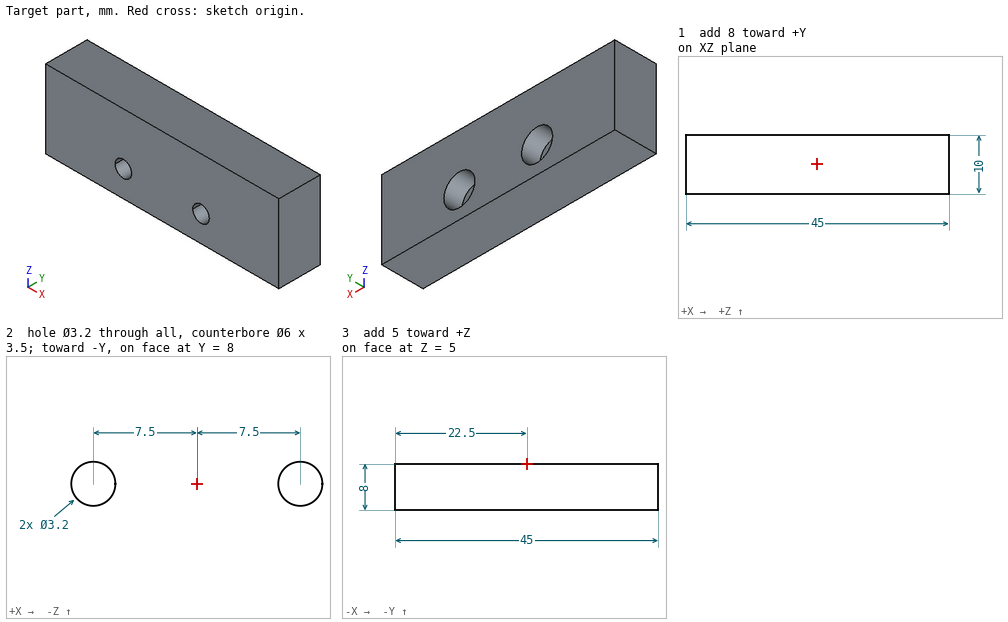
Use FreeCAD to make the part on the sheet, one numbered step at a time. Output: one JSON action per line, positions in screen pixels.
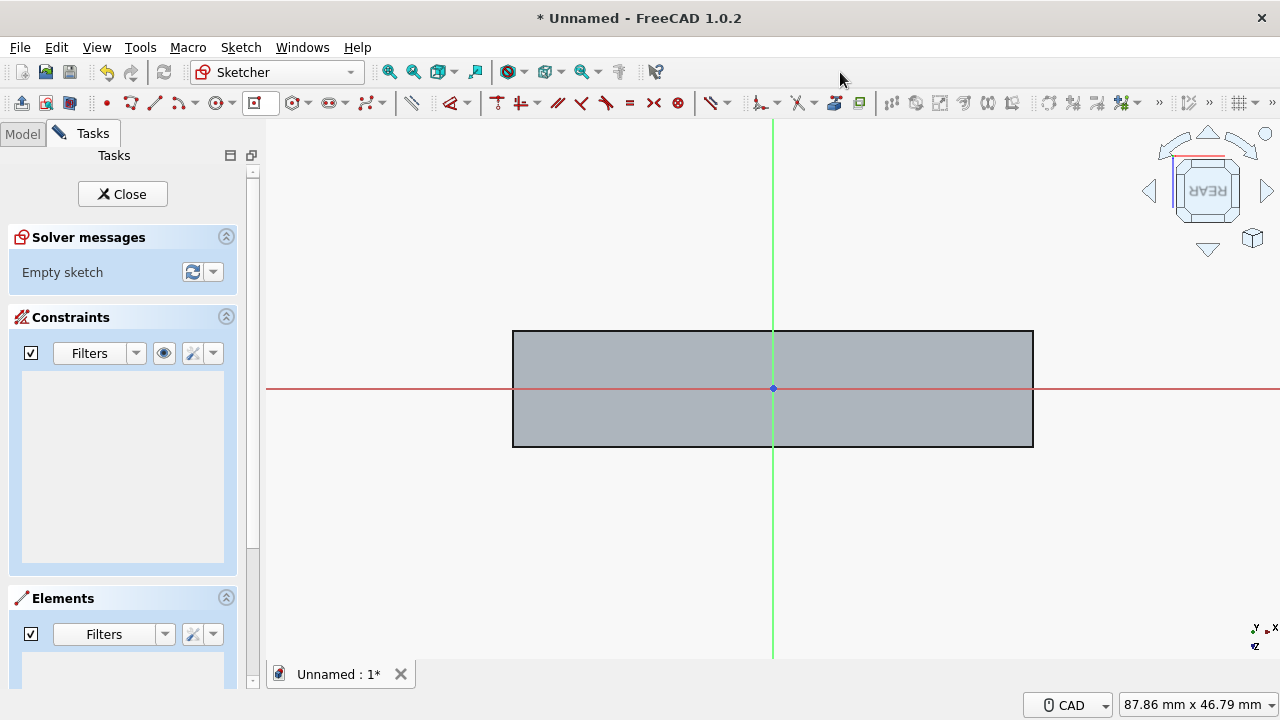
{"action": "scroll", "coordinate": [813, 389], "scroll_direction": "up", "scroll_amount": 5}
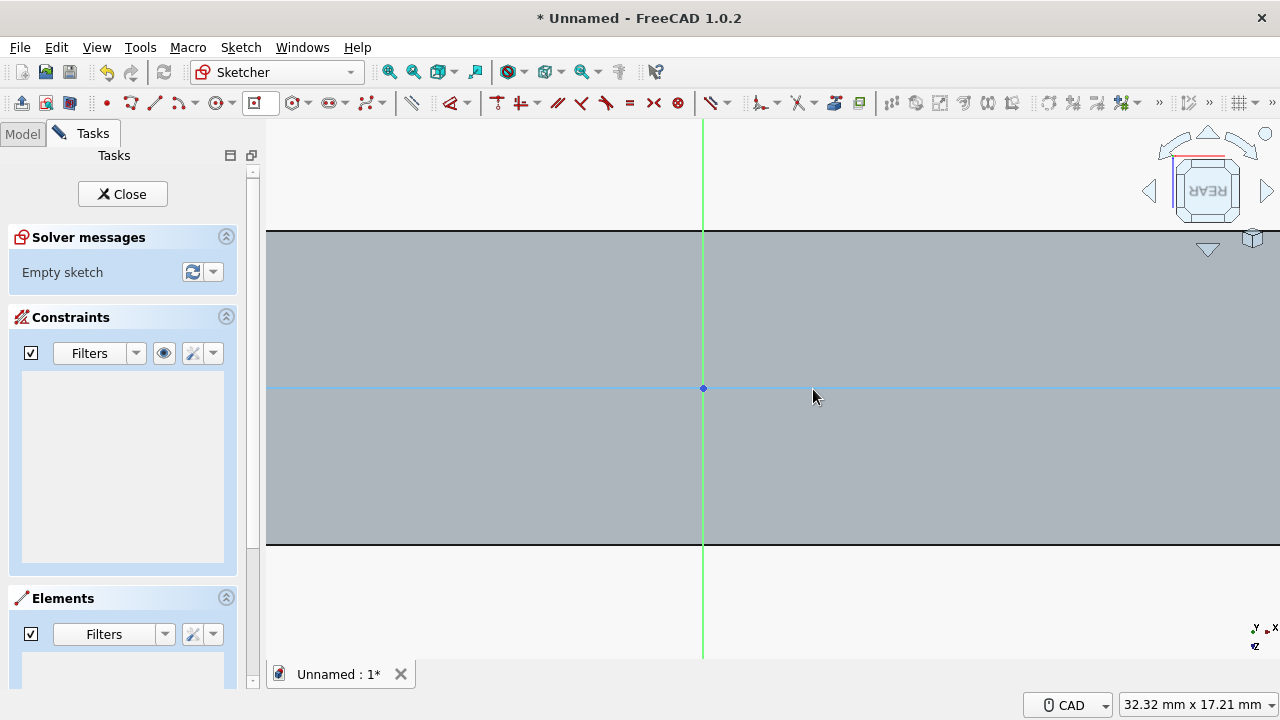
{"action": "key", "text": "g c"}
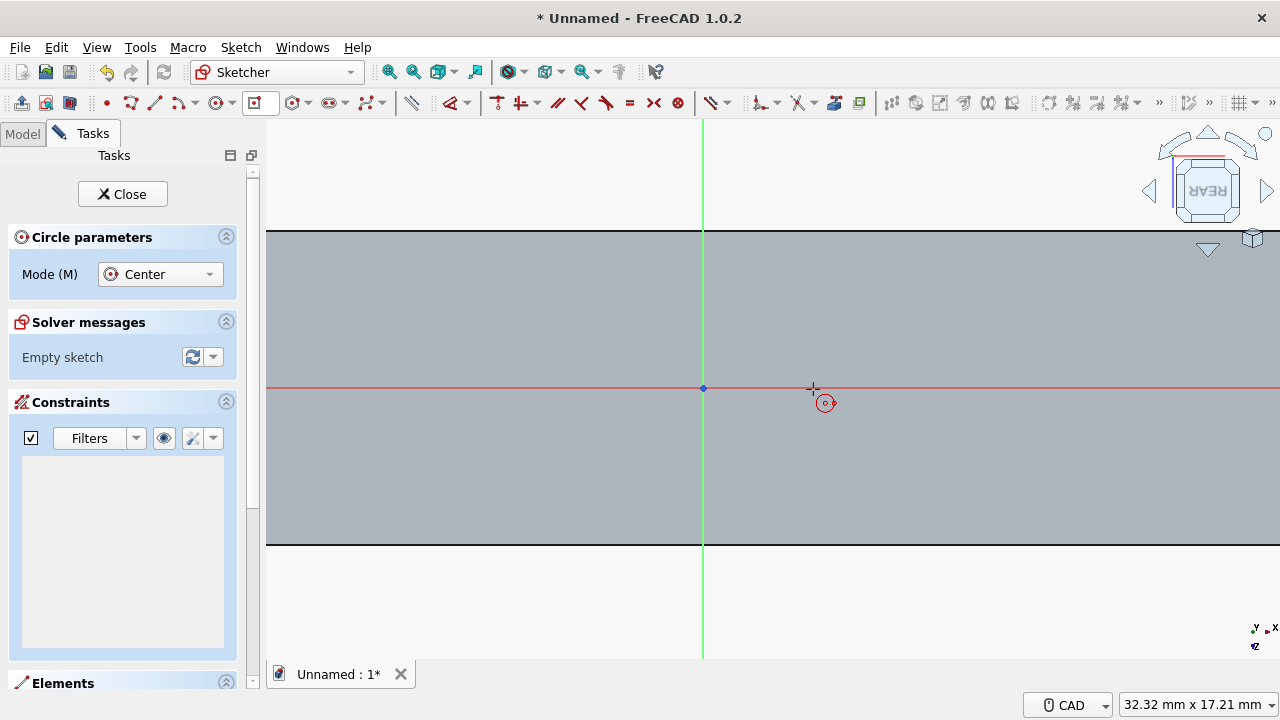
{"action": "left_click", "coordinate": [468, 388]}
{"action": "left_click", "coordinate": [504, 353]}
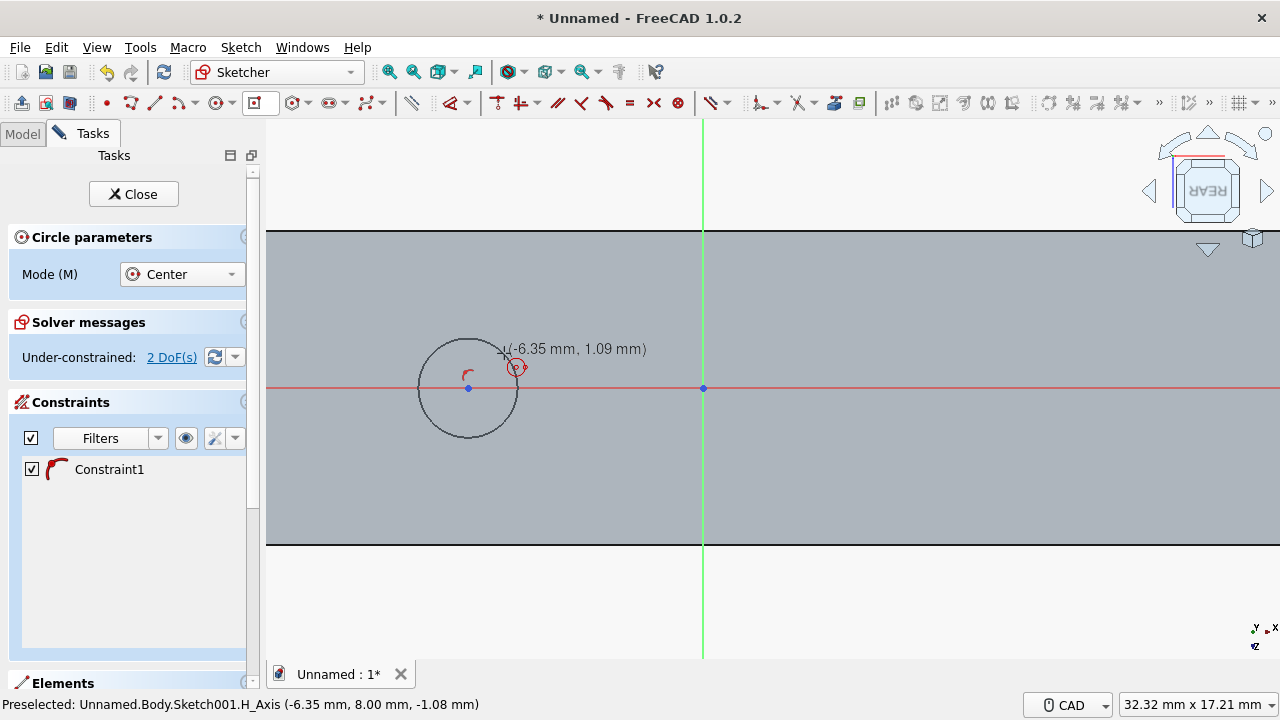
{"action": "left_click", "coordinate": [939, 388]}
{"action": "left_click", "coordinate": [974, 353]}
{"action": "key", "text": "Escape"}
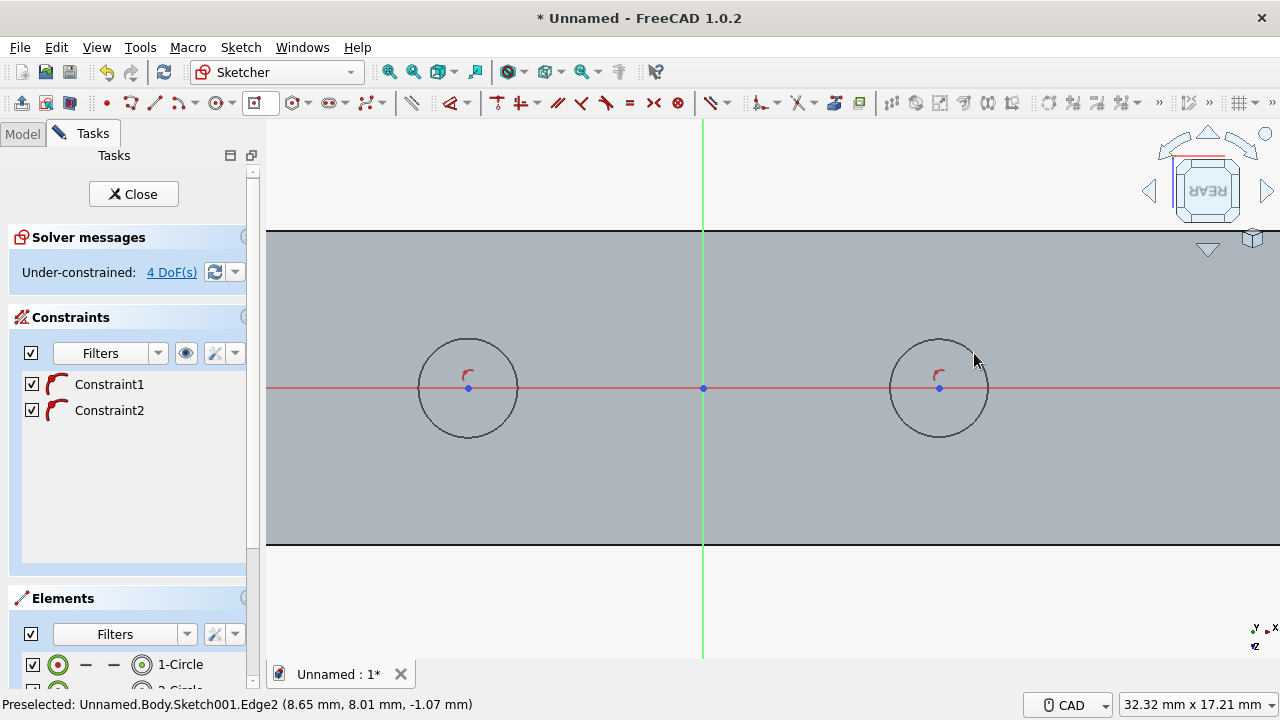
{"action": "left_click", "coordinate": [503, 353]}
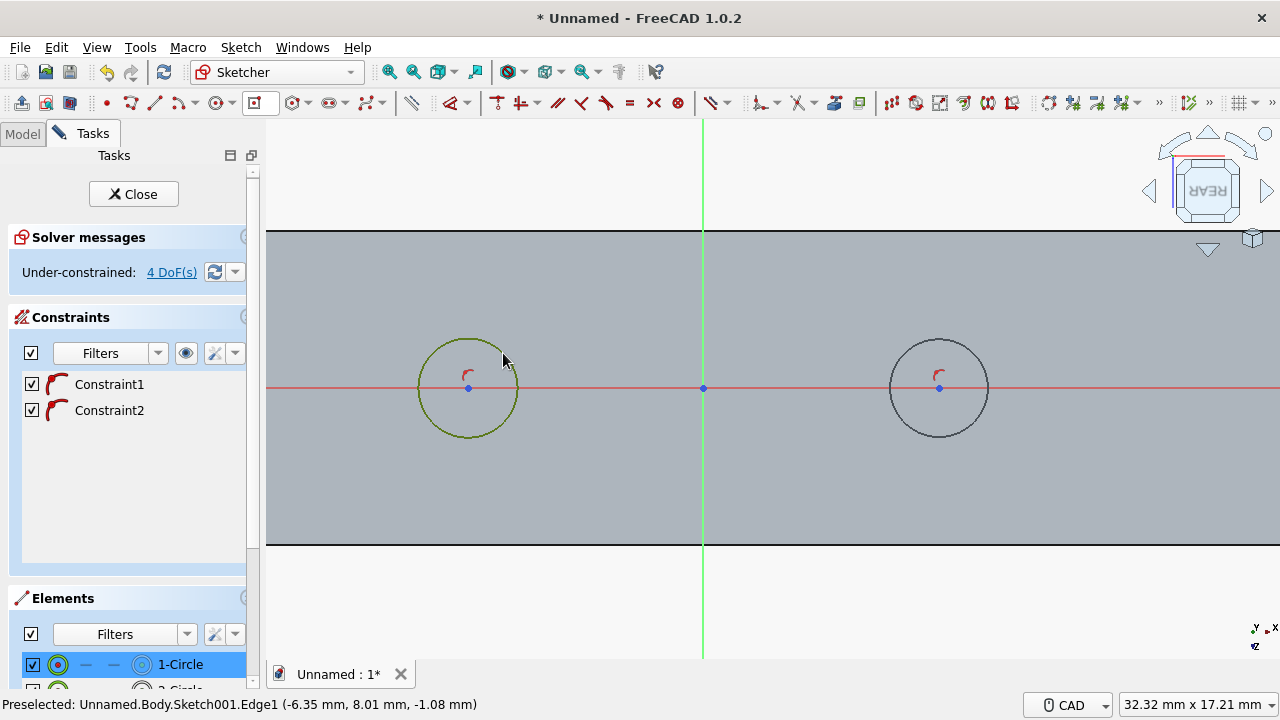
{"action": "left_click", "coordinate": [973, 353]}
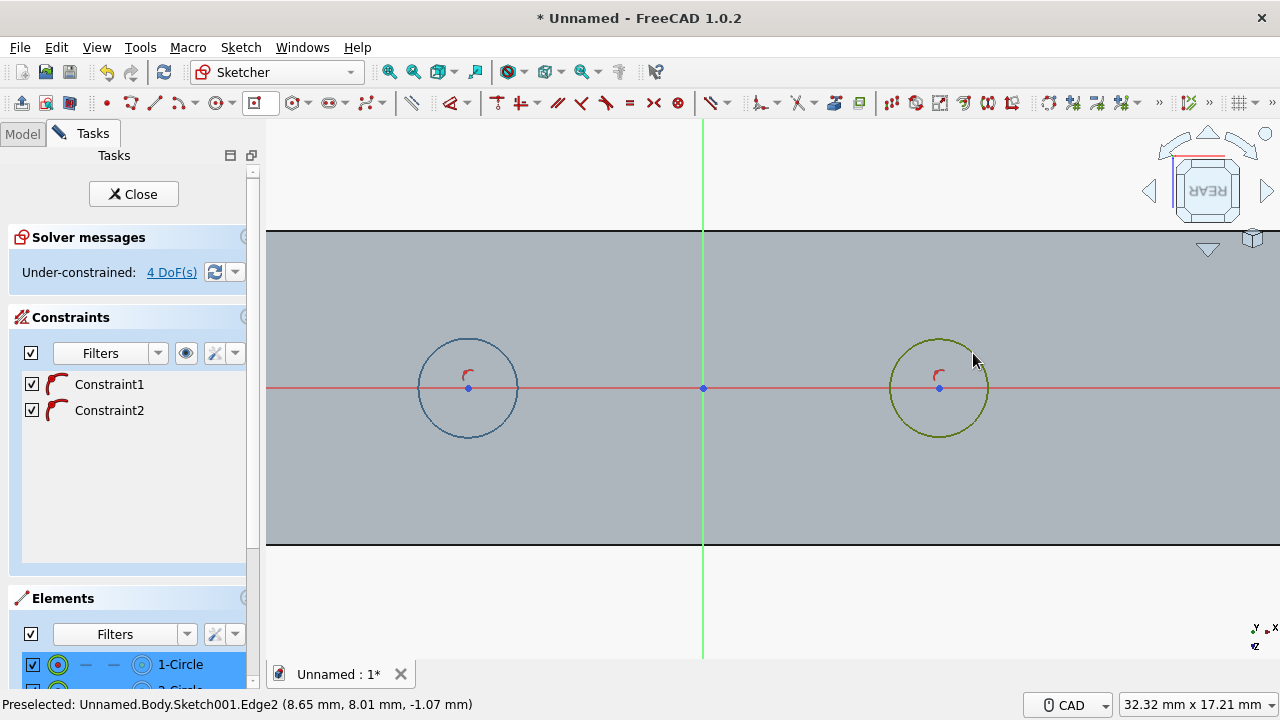
{"action": "left_click", "coordinate": [630, 104]}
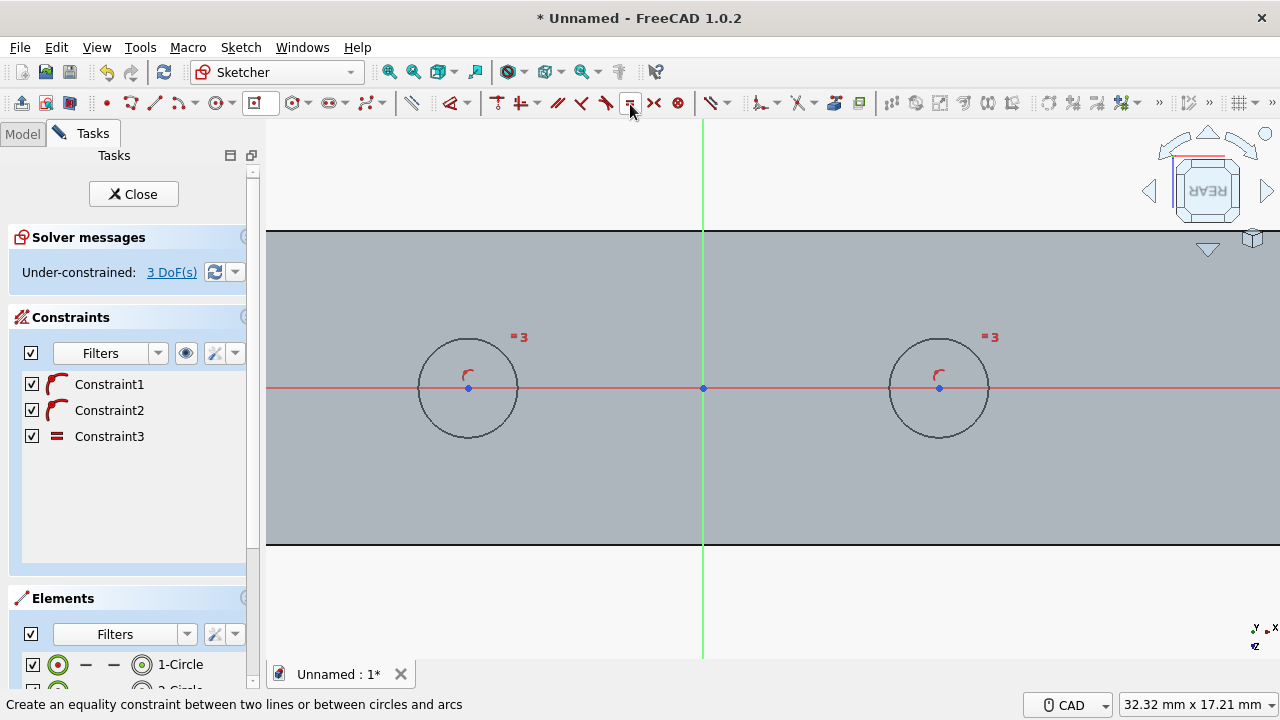
{"action": "left_click", "coordinate": [450, 104]}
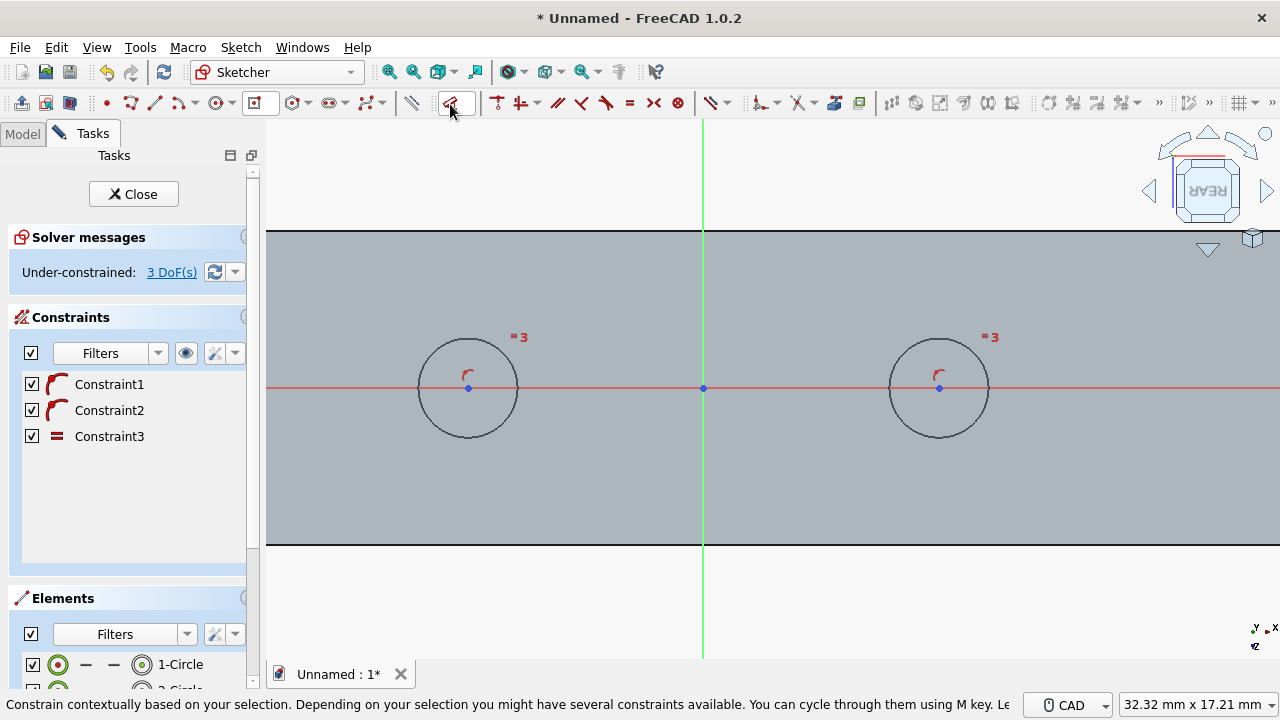
{"action": "left_click", "coordinate": [503, 353]}
{"action": "left_click", "coordinate": [526, 330]}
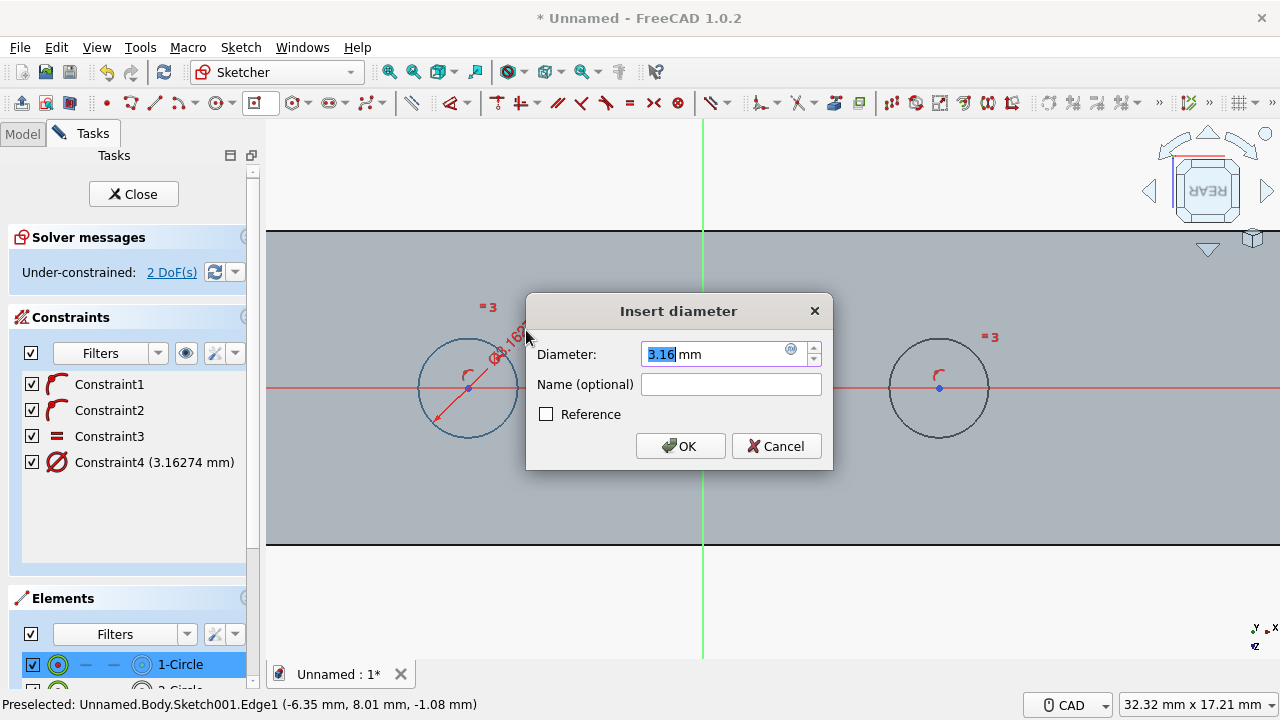
{"action": "type", "text": "3.2"}
{"action": "key", "text": "Return"}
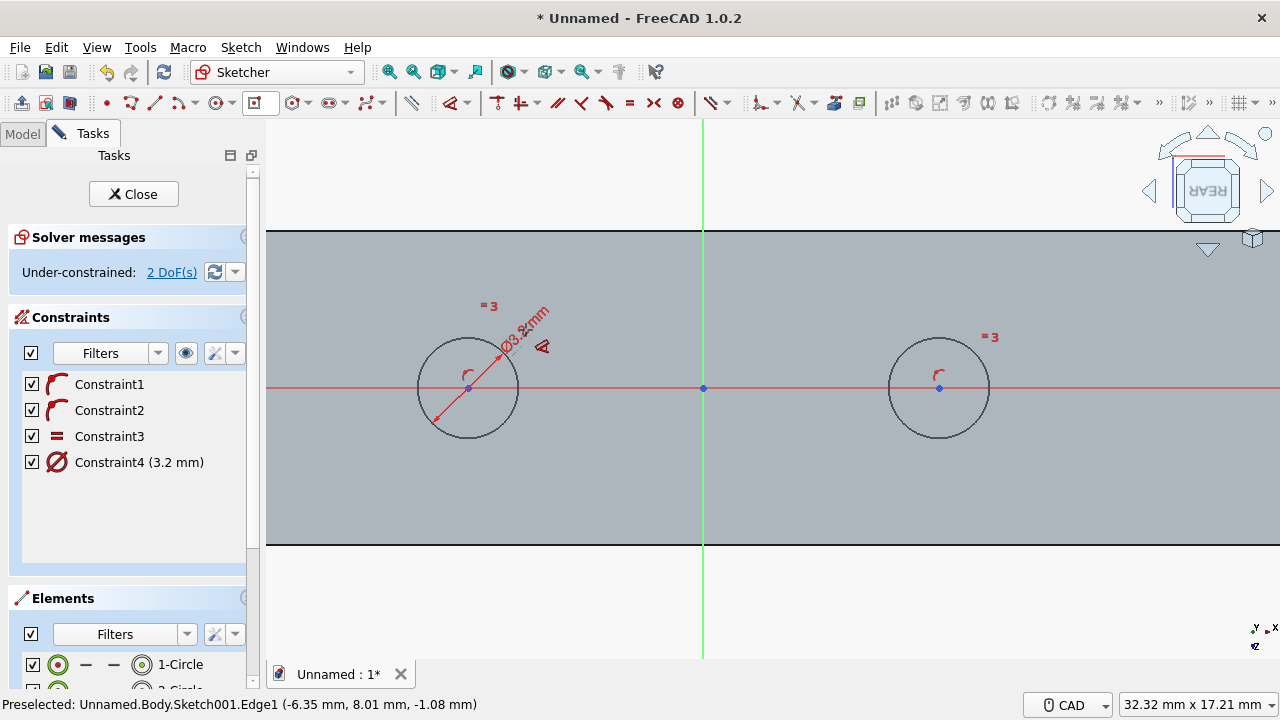
{"action": "left_click", "coordinate": [468, 388]}
{"action": "left_click", "coordinate": [586, 422]}